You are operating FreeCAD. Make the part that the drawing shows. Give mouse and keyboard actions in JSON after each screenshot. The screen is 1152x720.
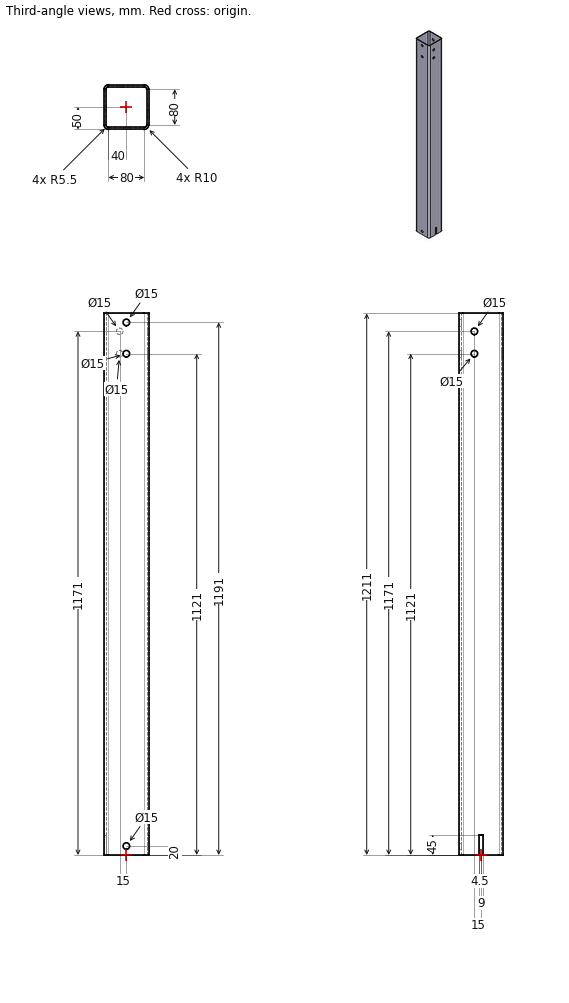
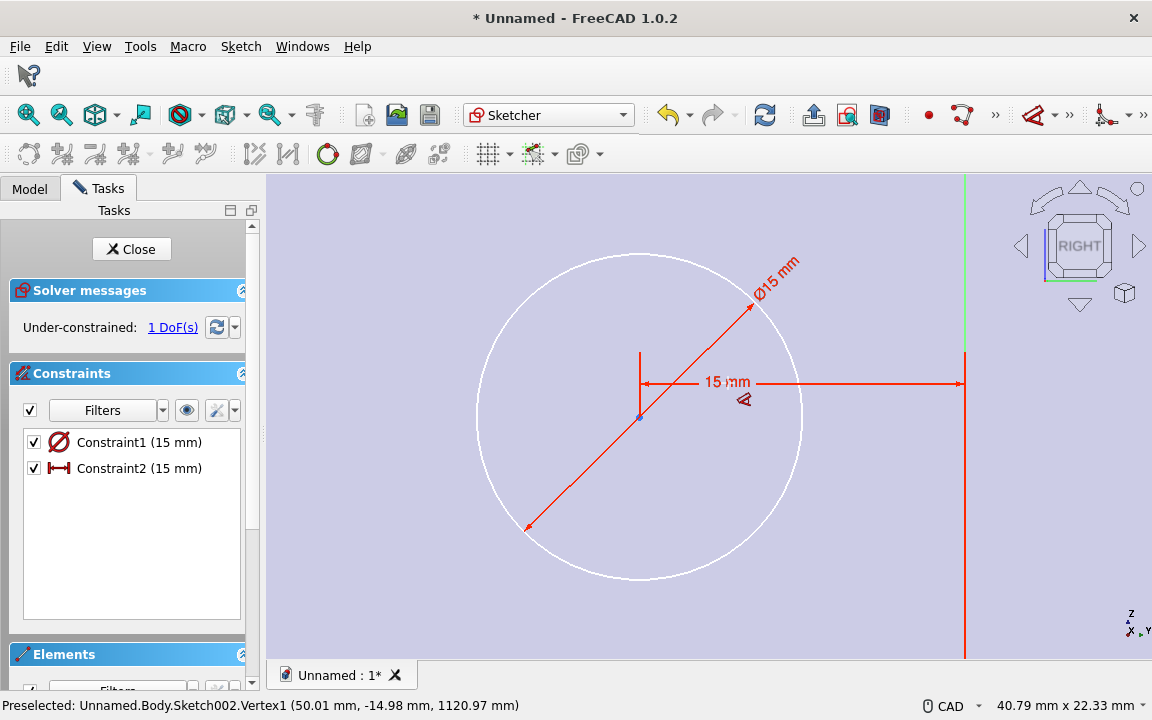
{"action": "left_click", "coordinate": [640, 417]}
{"action": "left_click", "coordinate": [606, 524]}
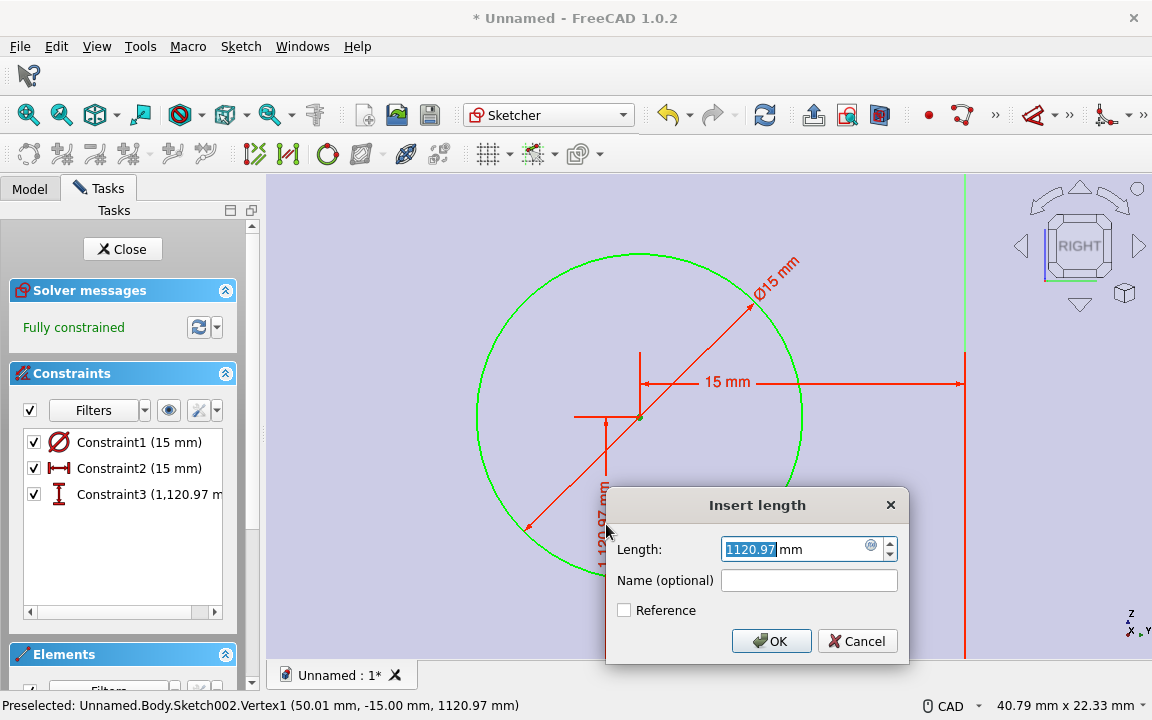
{"action": "type", "text": "1121"}
{"action": "key", "text": "Return"}
{"action": "key", "text": "Escape"}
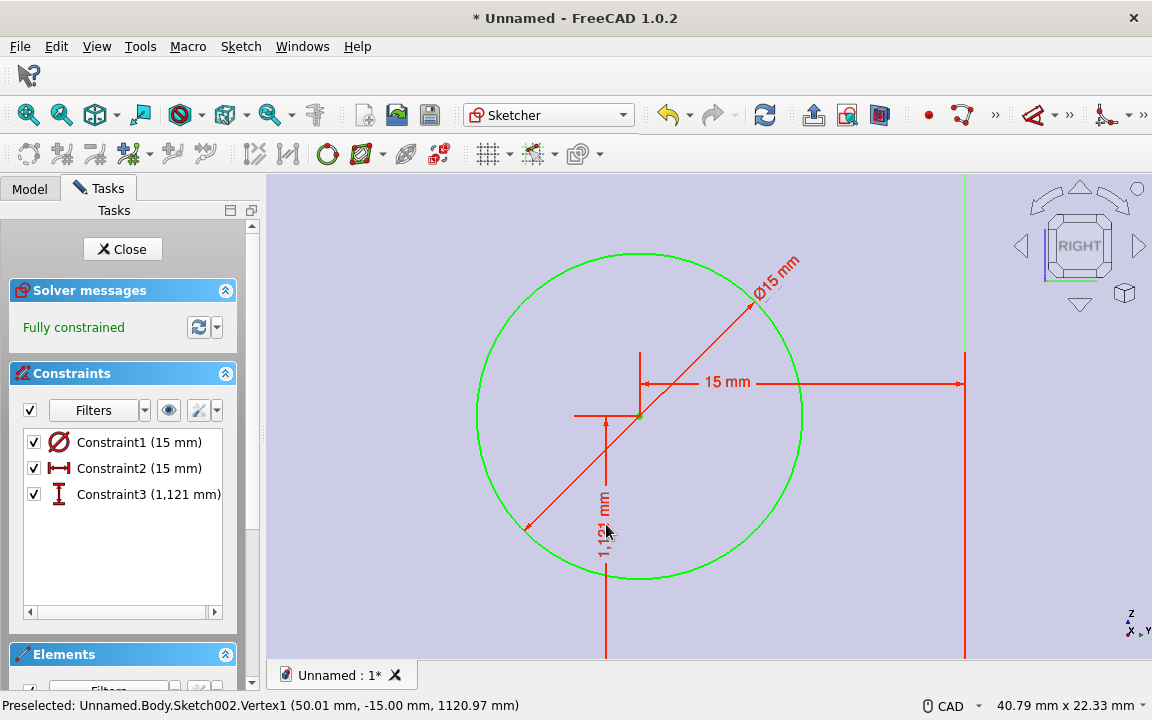
{"action": "left_click", "coordinate": [123, 249]}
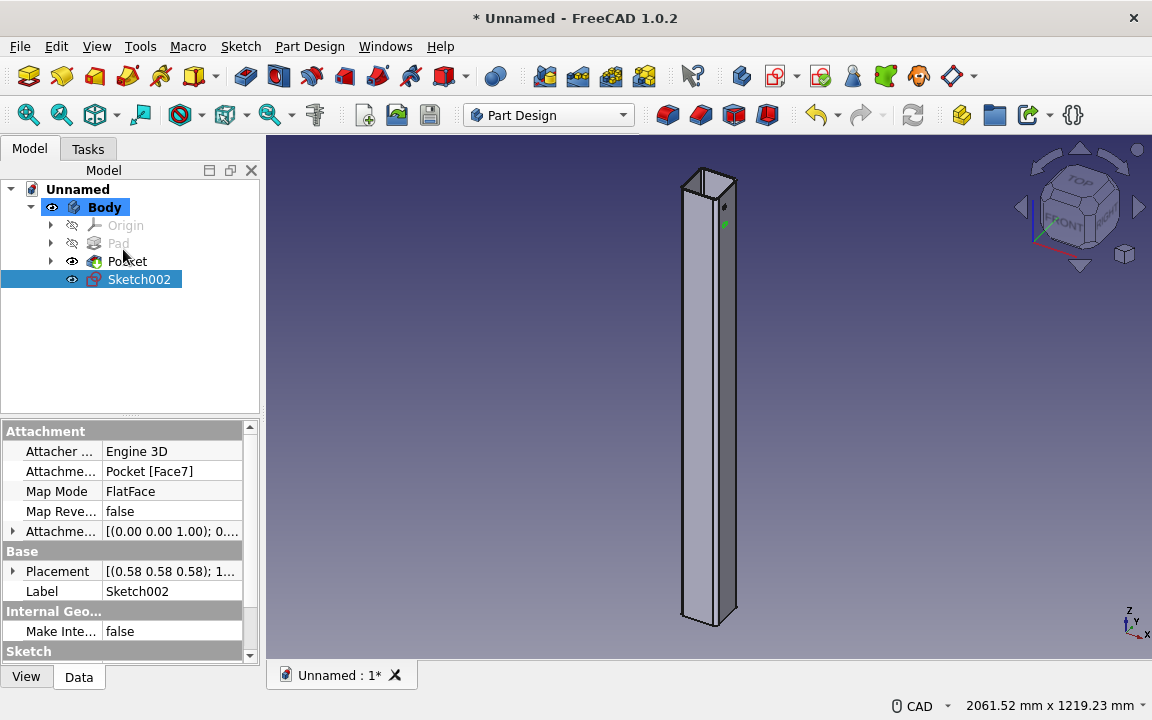
{"action": "left_click", "coordinate": [246, 76]}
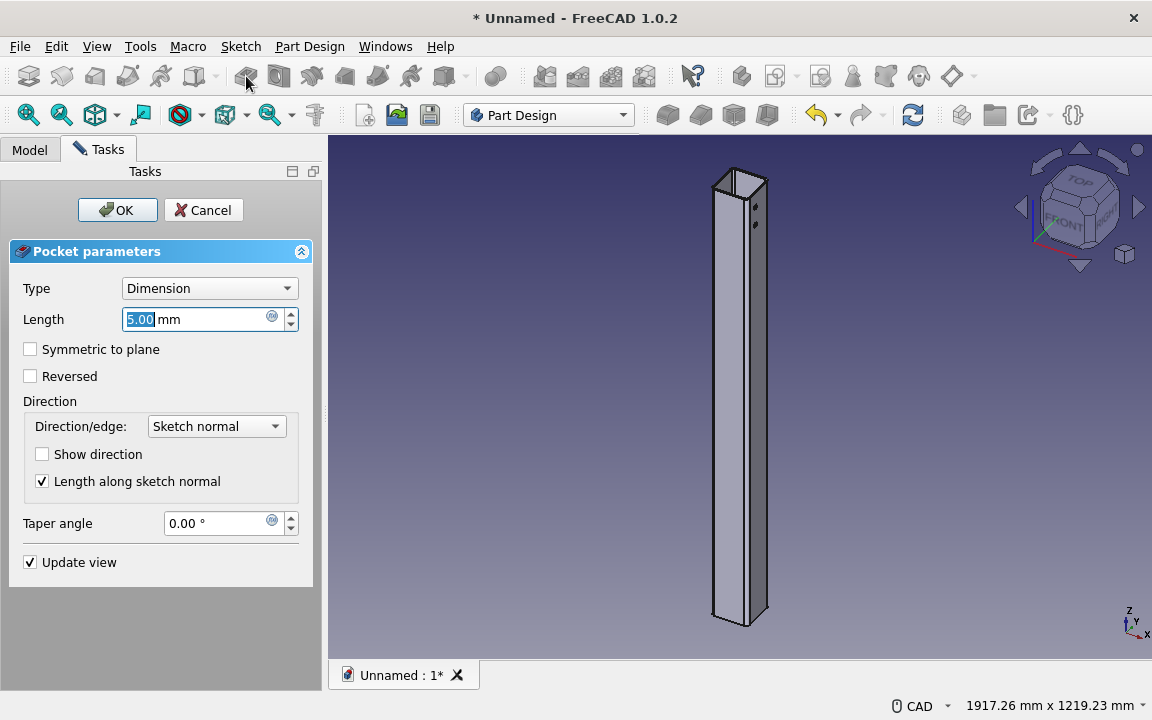
{"action": "left_click", "coordinate": [210, 288]}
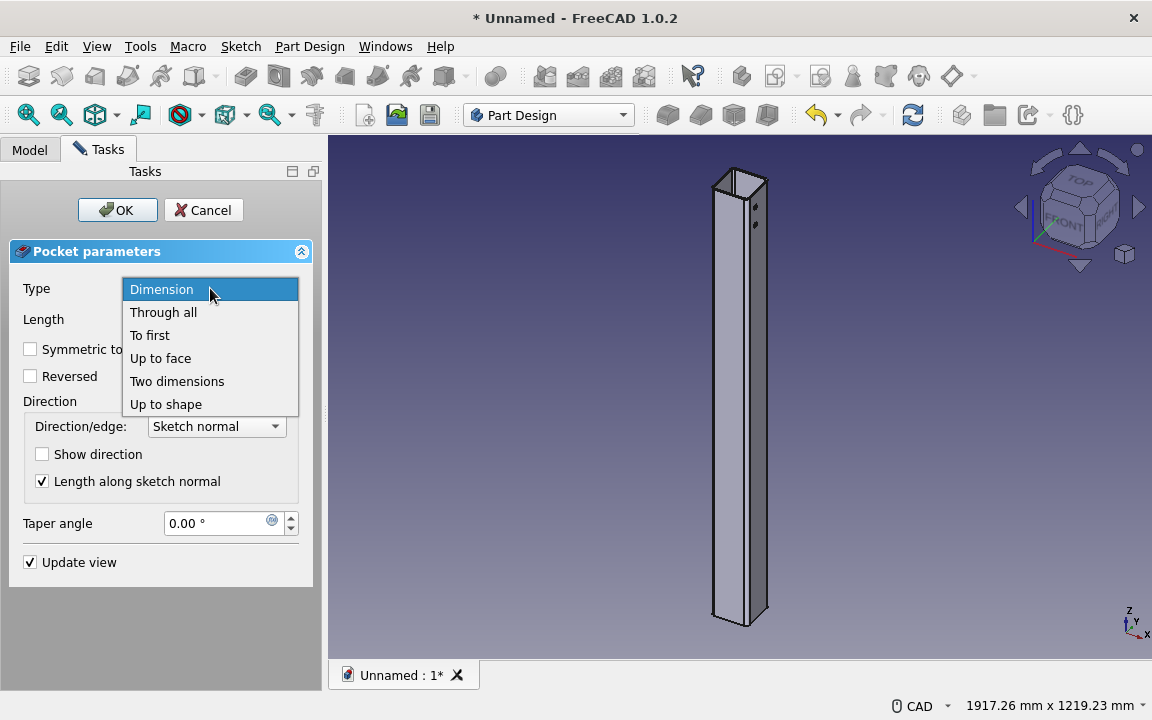
{"action": "left_click", "coordinate": [208, 336]}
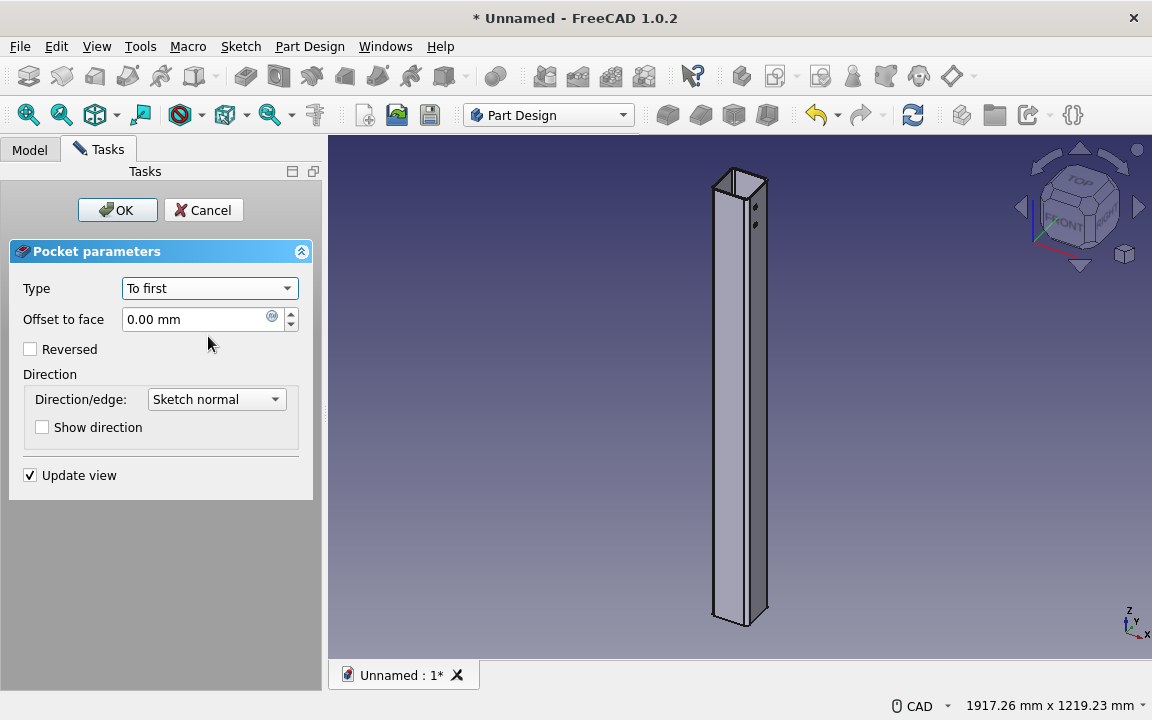
{"action": "left_click", "coordinate": [118, 210]}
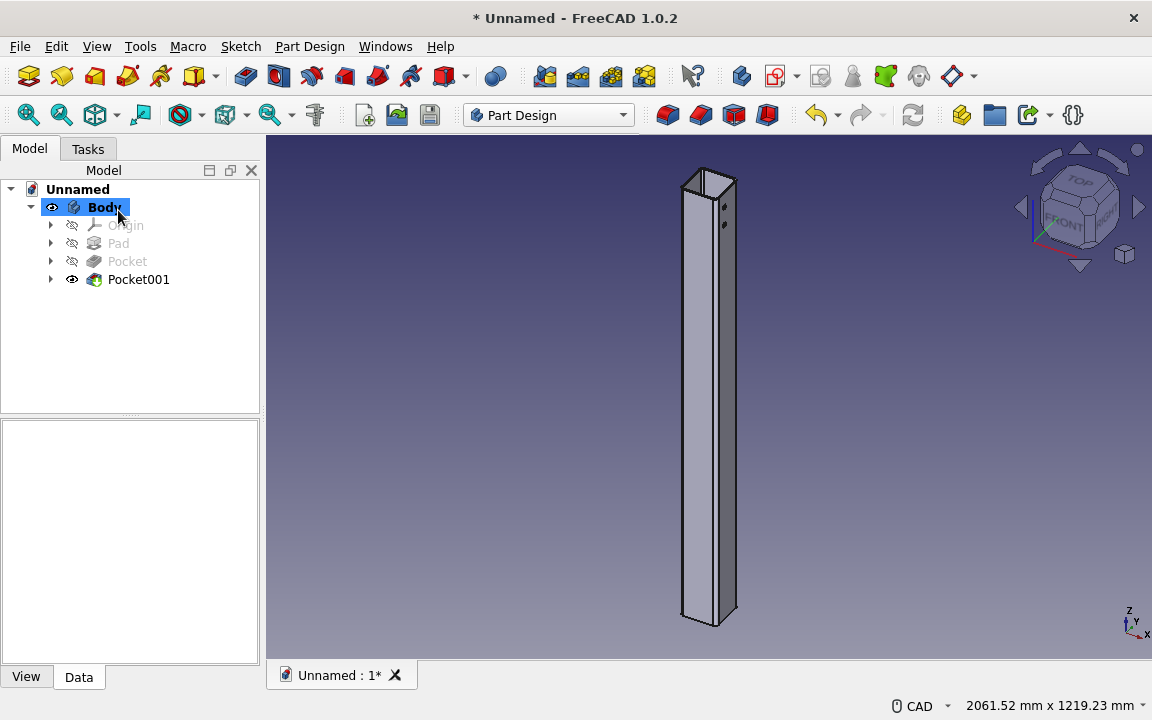
{"action": "left_click", "coordinate": [698, 224]}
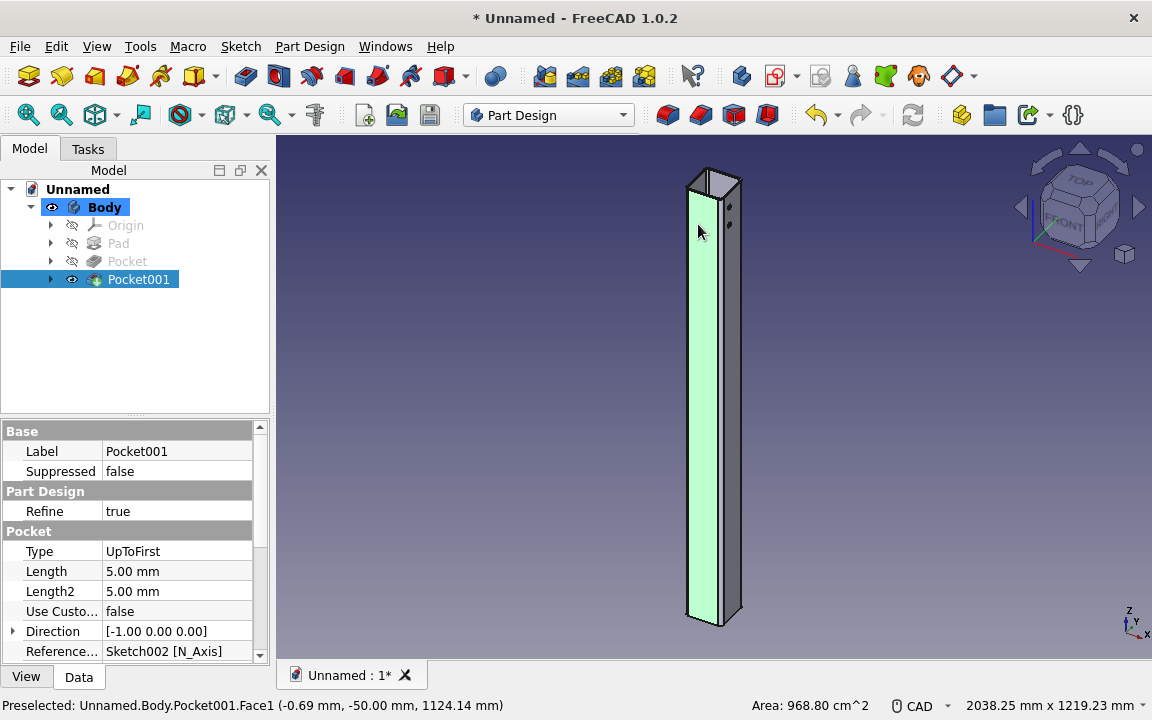
{"action": "left_click", "coordinate": [774, 76]}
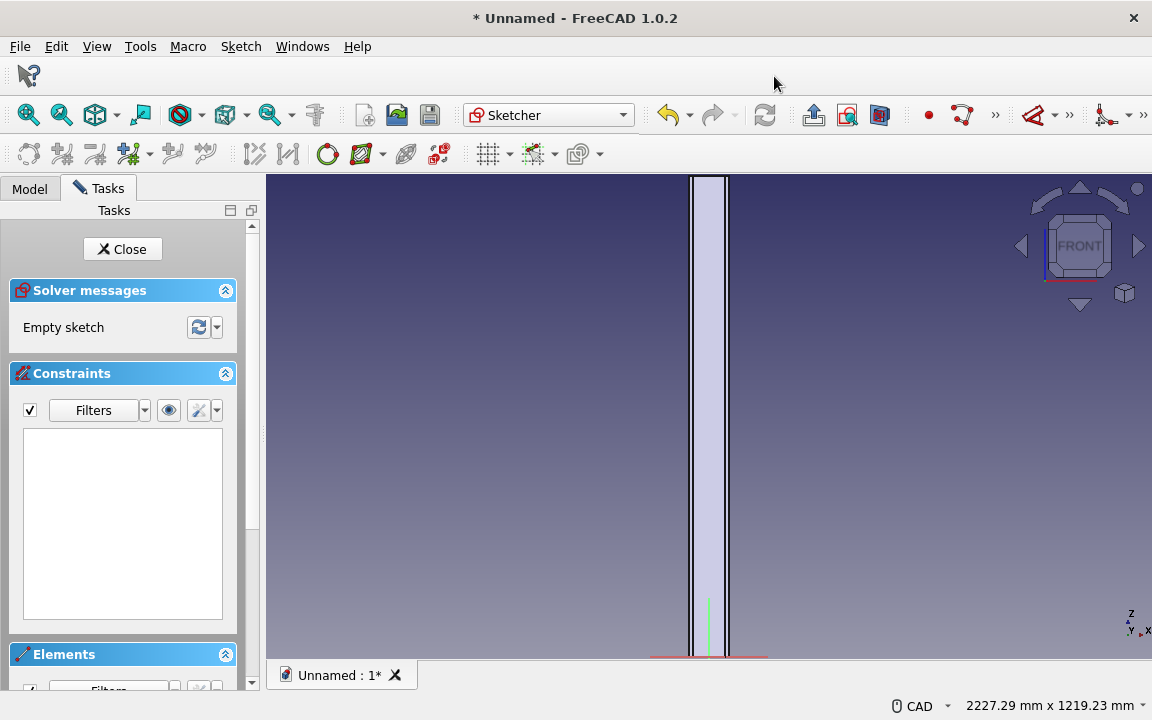
{"action": "scroll", "coordinate": [640, 416], "scroll_direction": "down", "scroll_amount": 5}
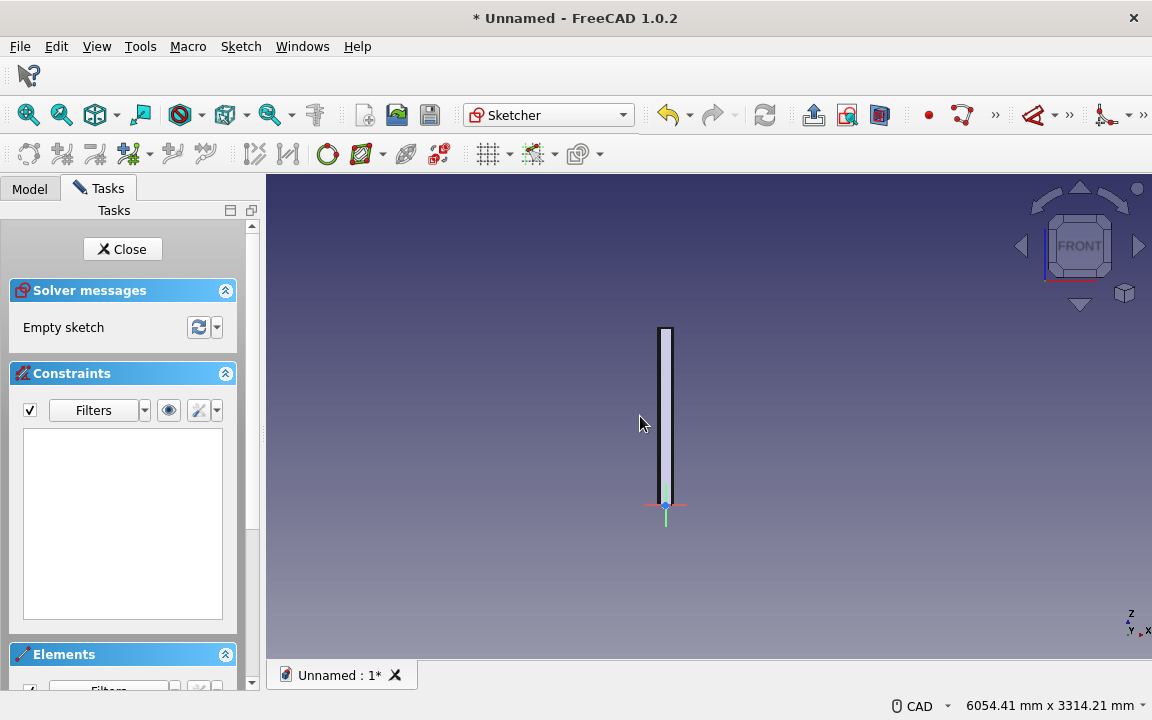
{"action": "scroll", "coordinate": [667, 326], "scroll_direction": "up", "scroll_amount": 15}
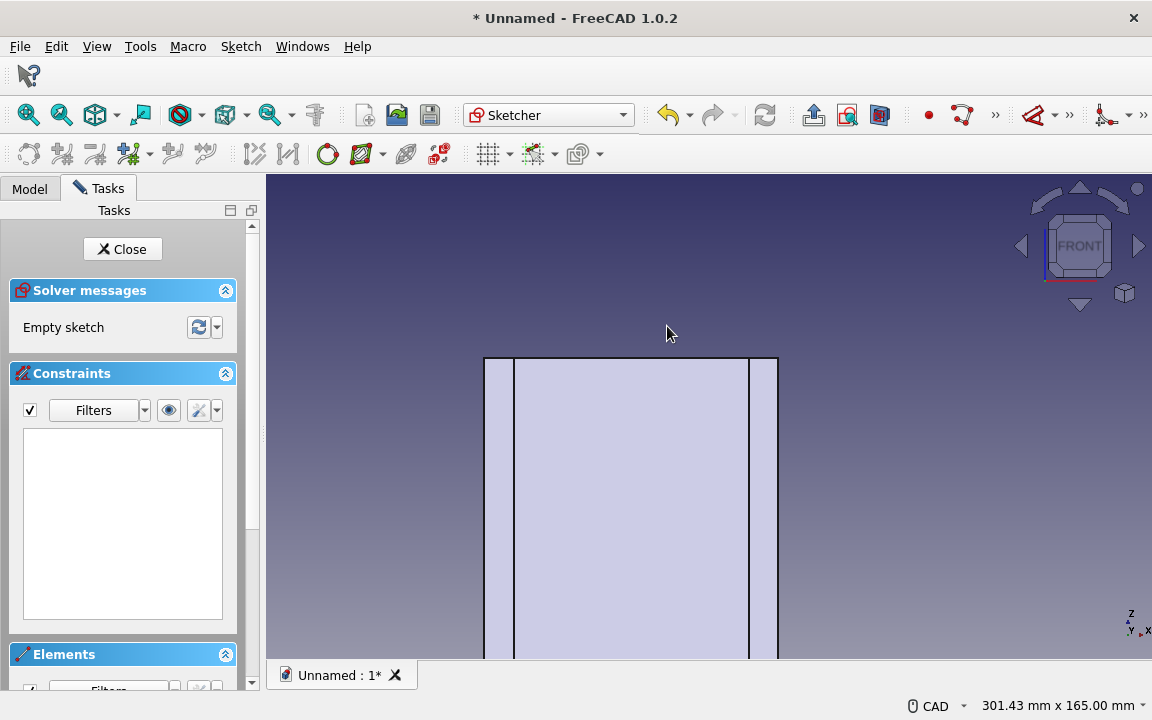
{"action": "scroll", "coordinate": [630, 417], "scroll_direction": "up", "scroll_amount": 10}